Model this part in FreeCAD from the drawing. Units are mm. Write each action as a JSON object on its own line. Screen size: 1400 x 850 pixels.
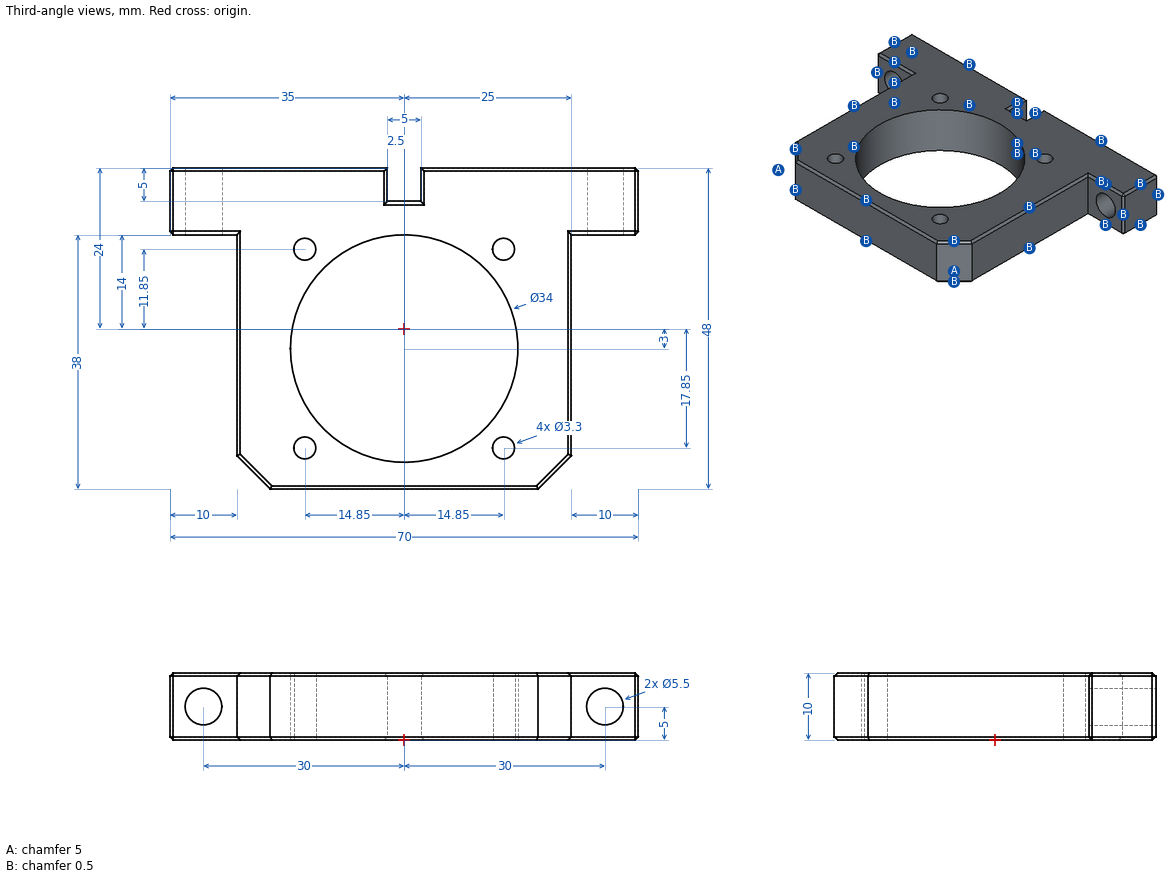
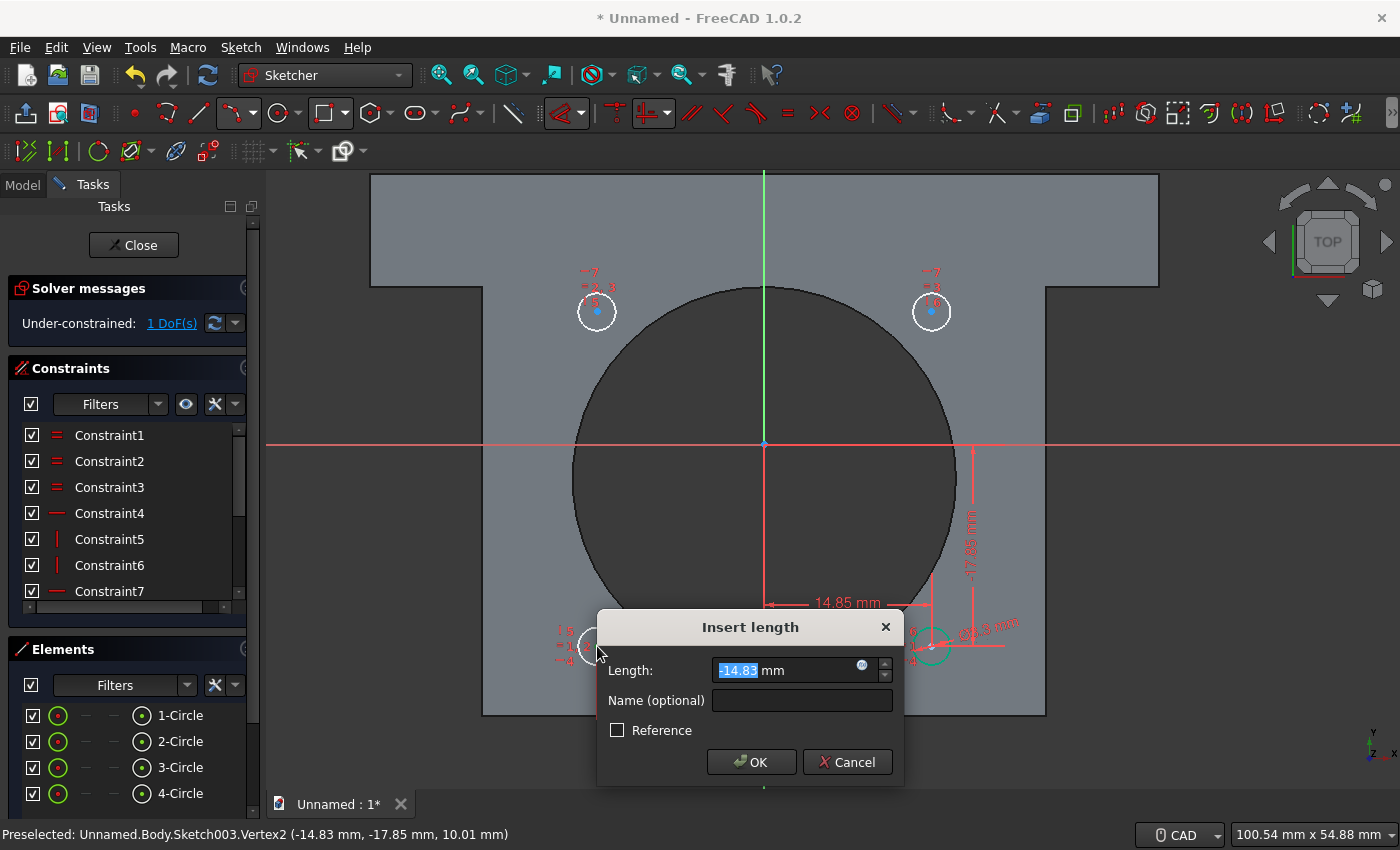
{"action": "type", "text": "-14.85"}
{"action": "key", "text": "Return"}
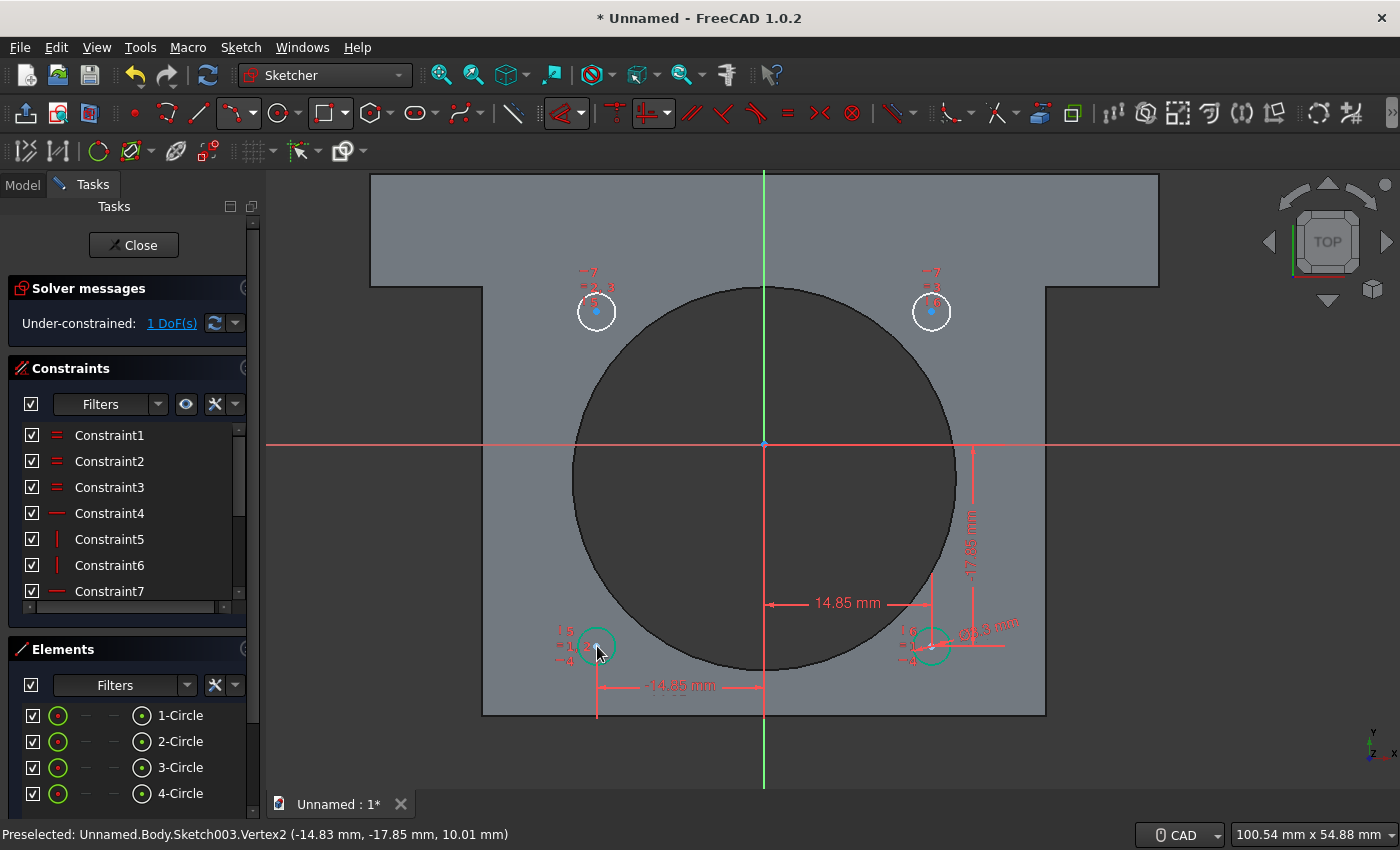
{"action": "left_click", "coordinate": [597, 312]}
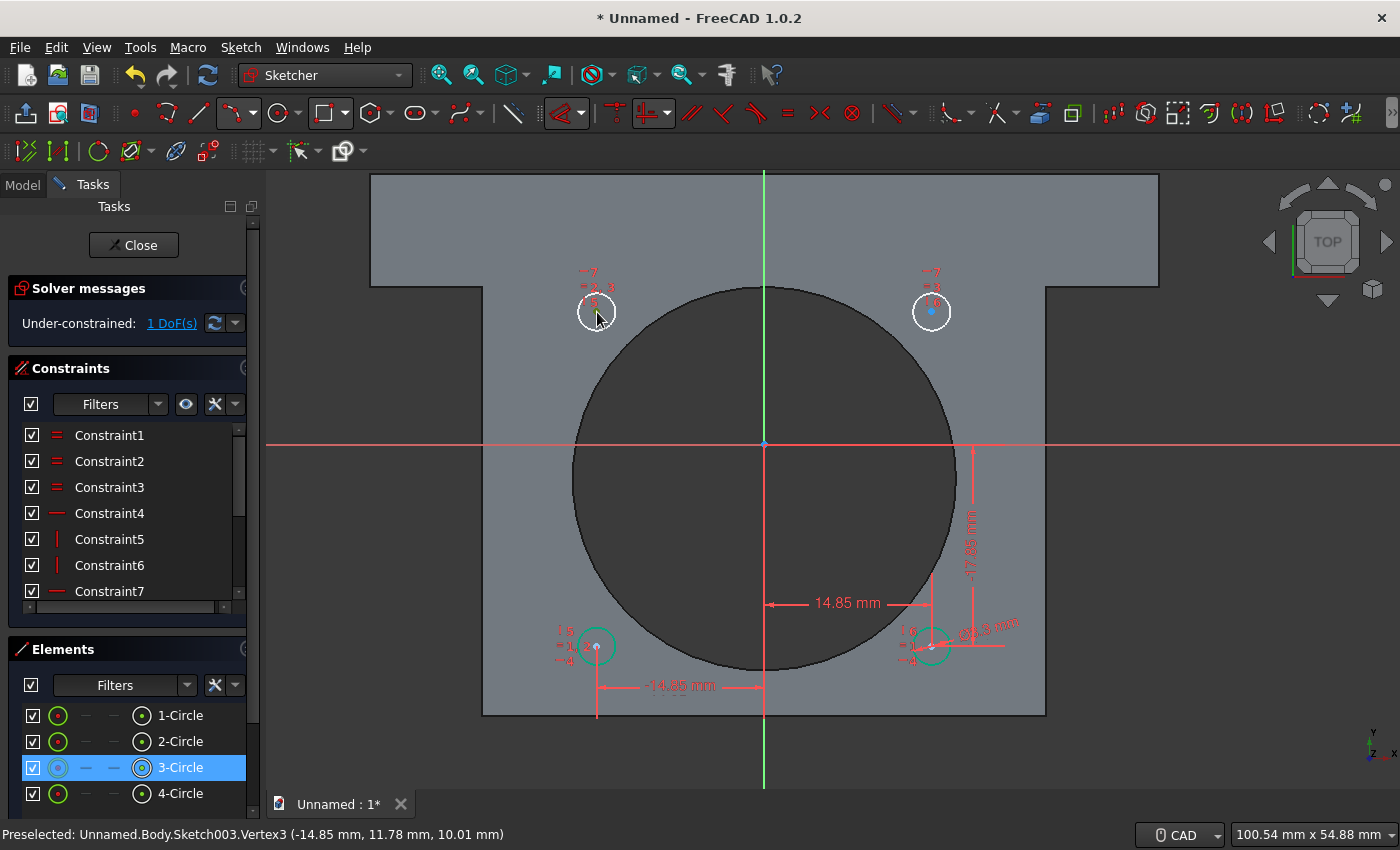
{"action": "left_click", "coordinate": [584, 114]}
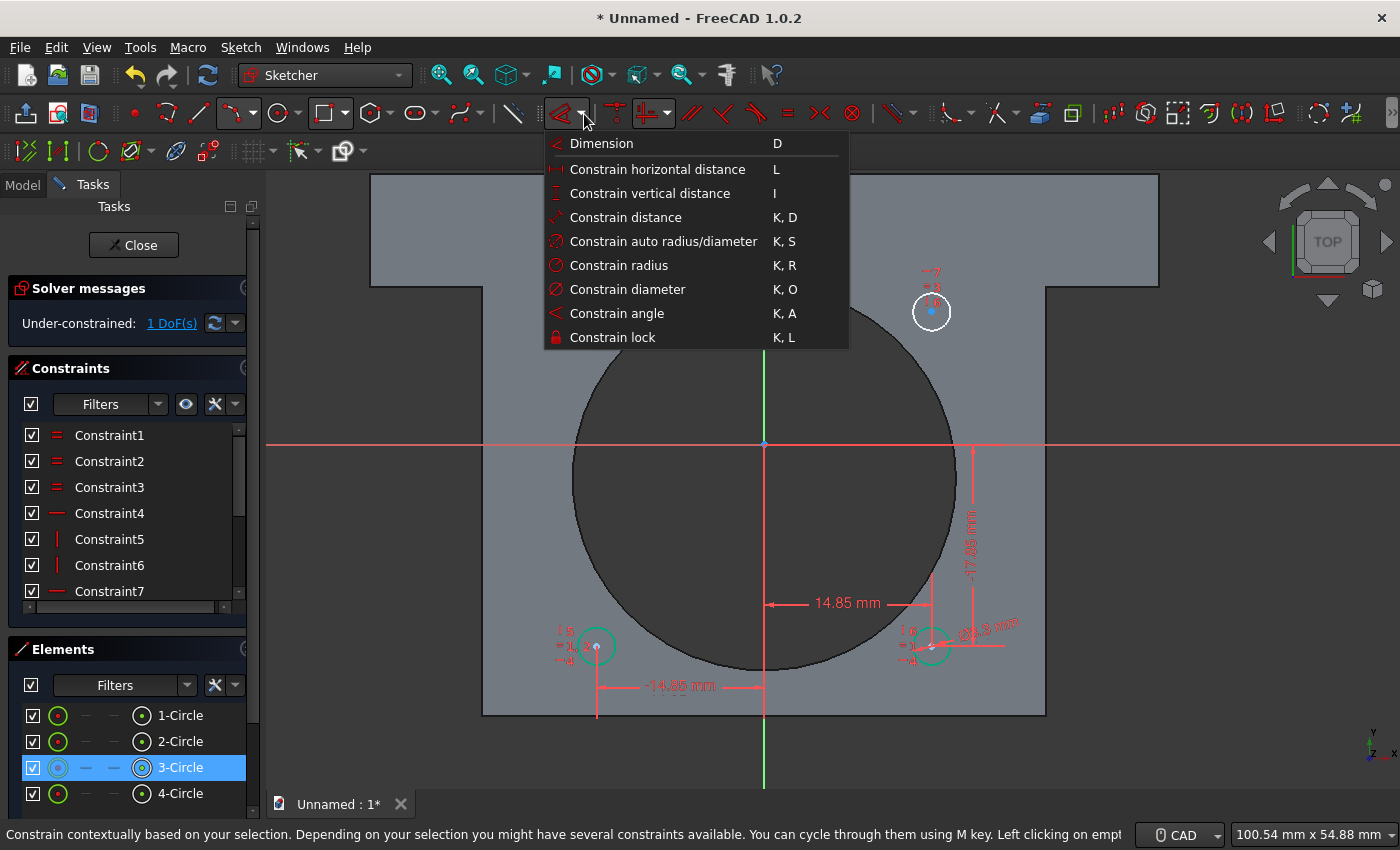
{"action": "left_click", "coordinate": [697, 193]}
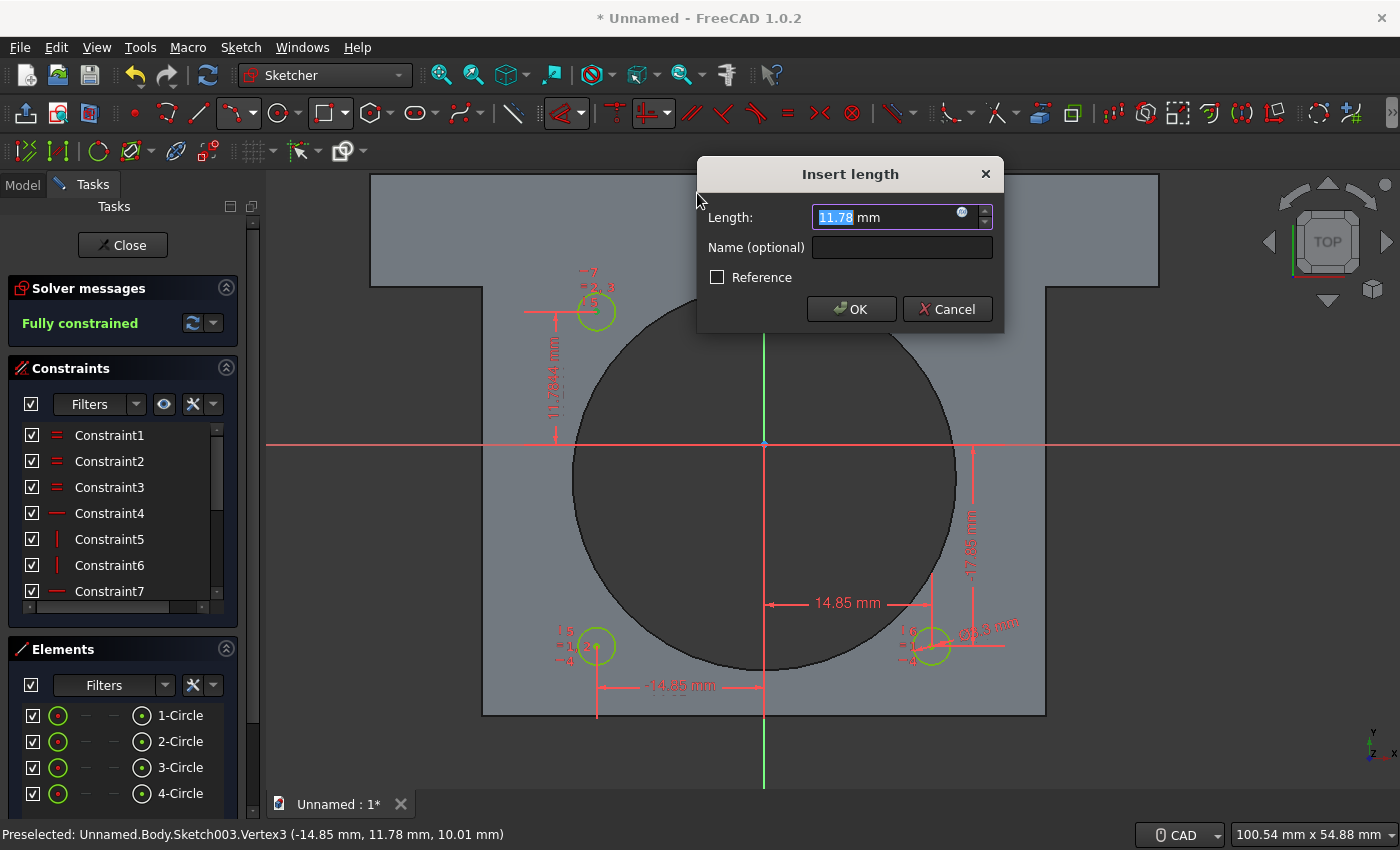
{"action": "type", "text": "11.85"}
{"action": "key", "text": "Return"}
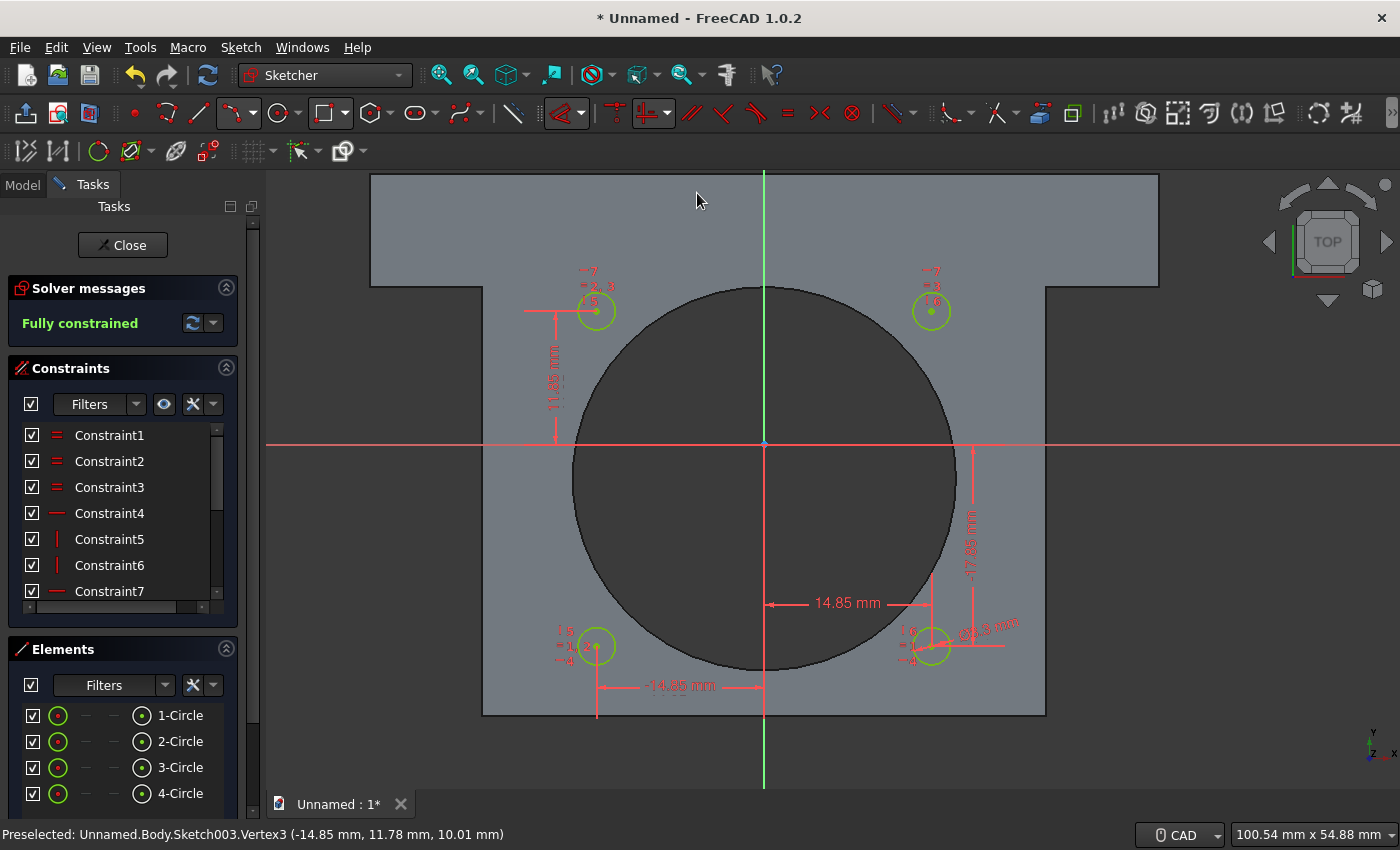
{"action": "left_click", "coordinate": [123, 245]}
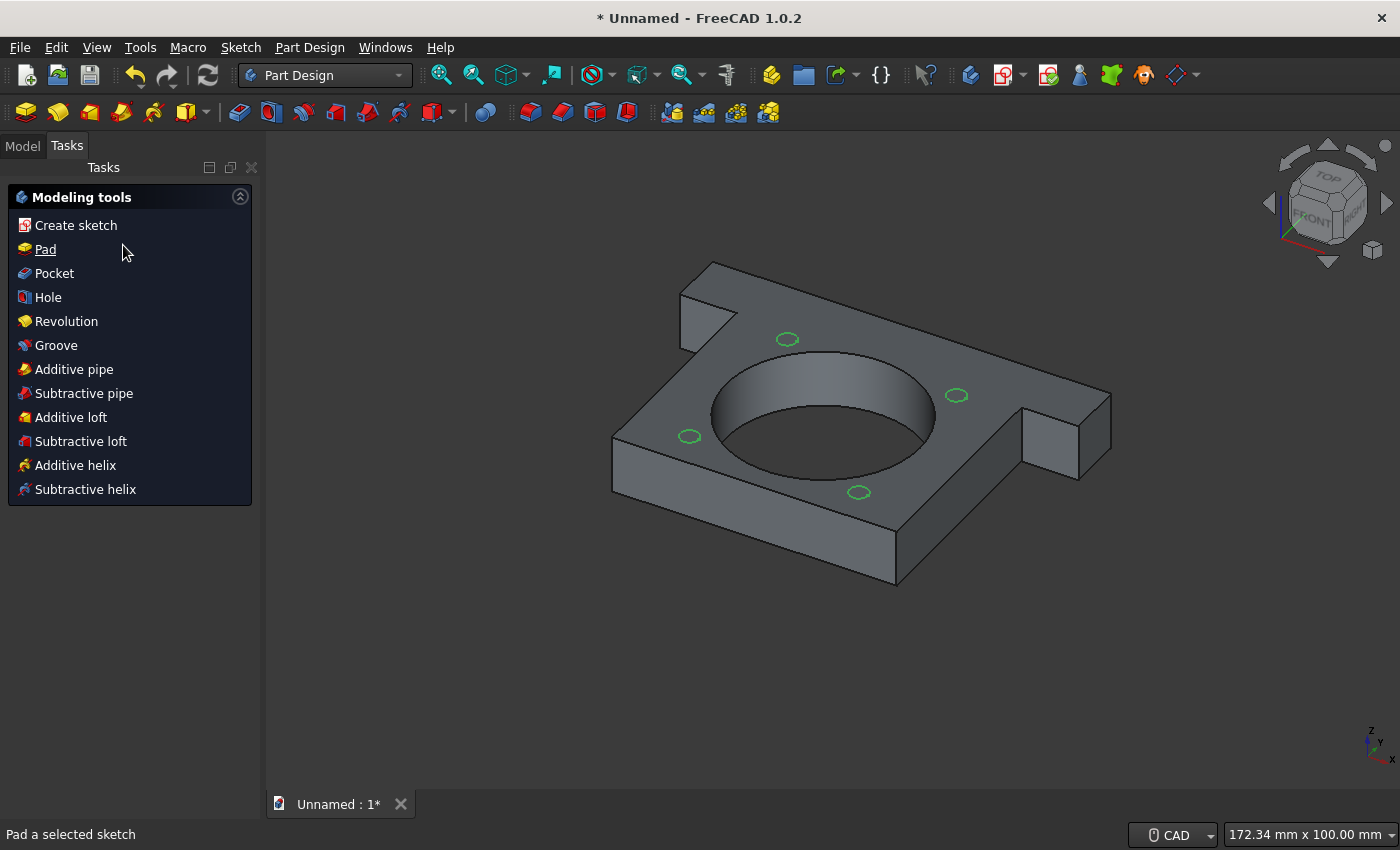
{"action": "left_click", "coordinate": [240, 112]}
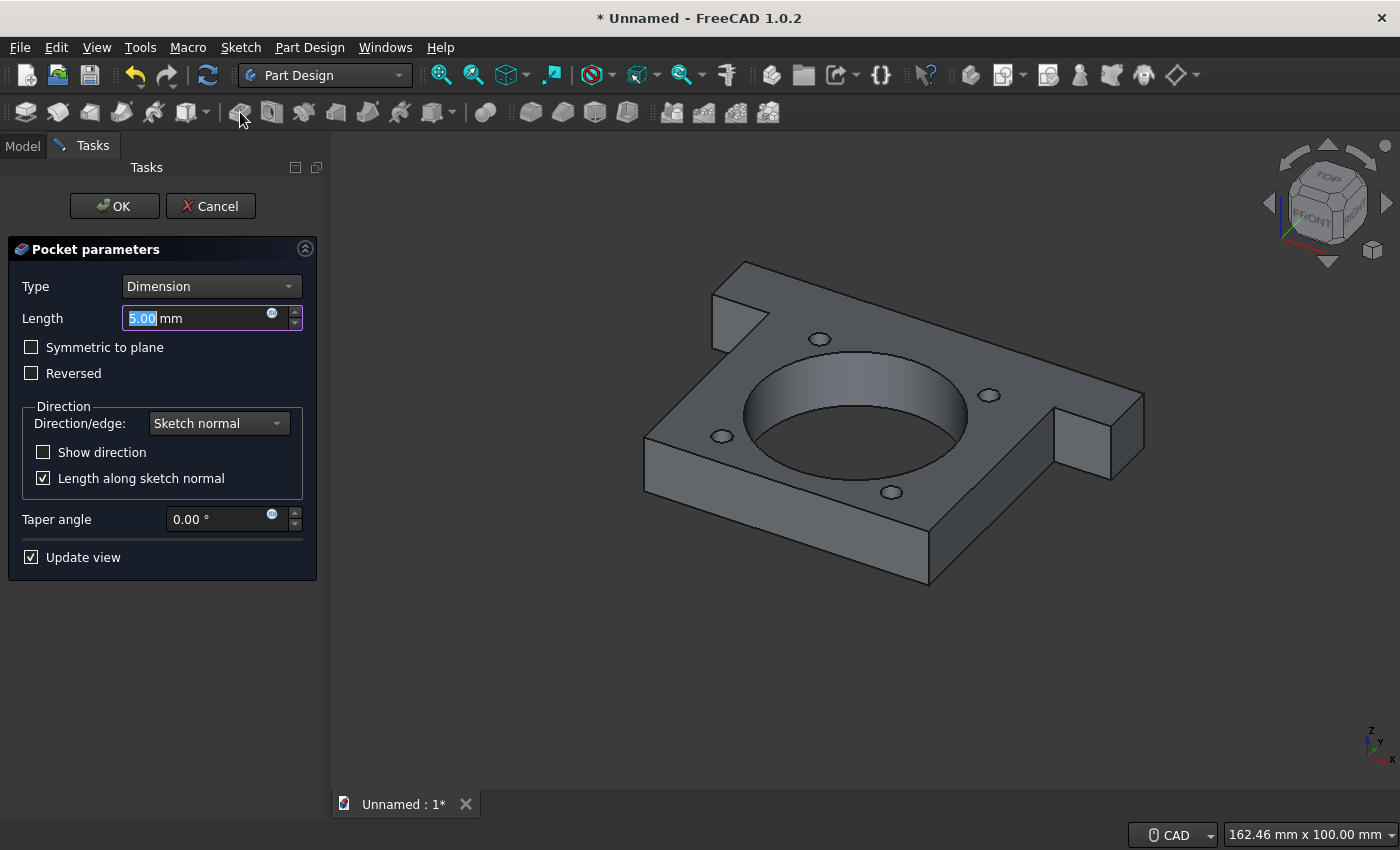
{"action": "left_click", "coordinate": [212, 286]}